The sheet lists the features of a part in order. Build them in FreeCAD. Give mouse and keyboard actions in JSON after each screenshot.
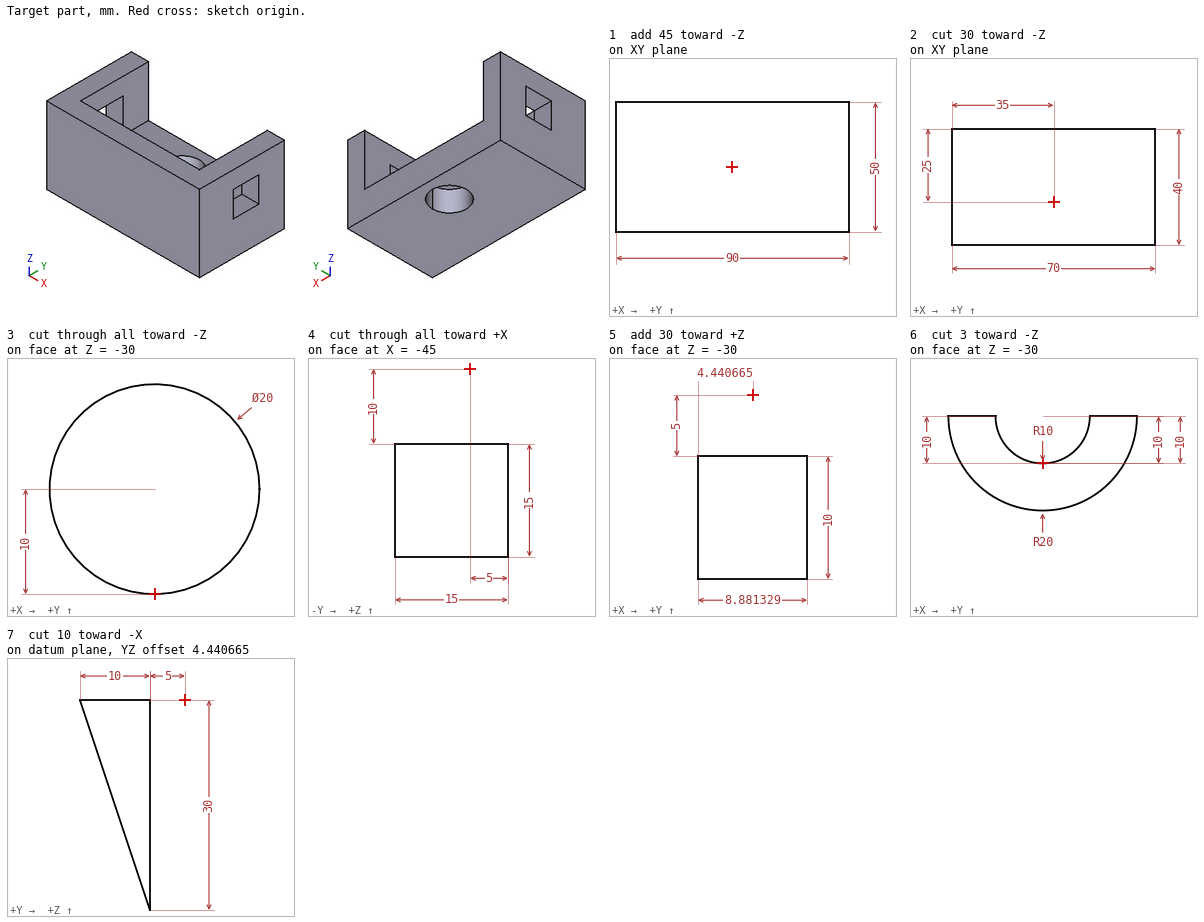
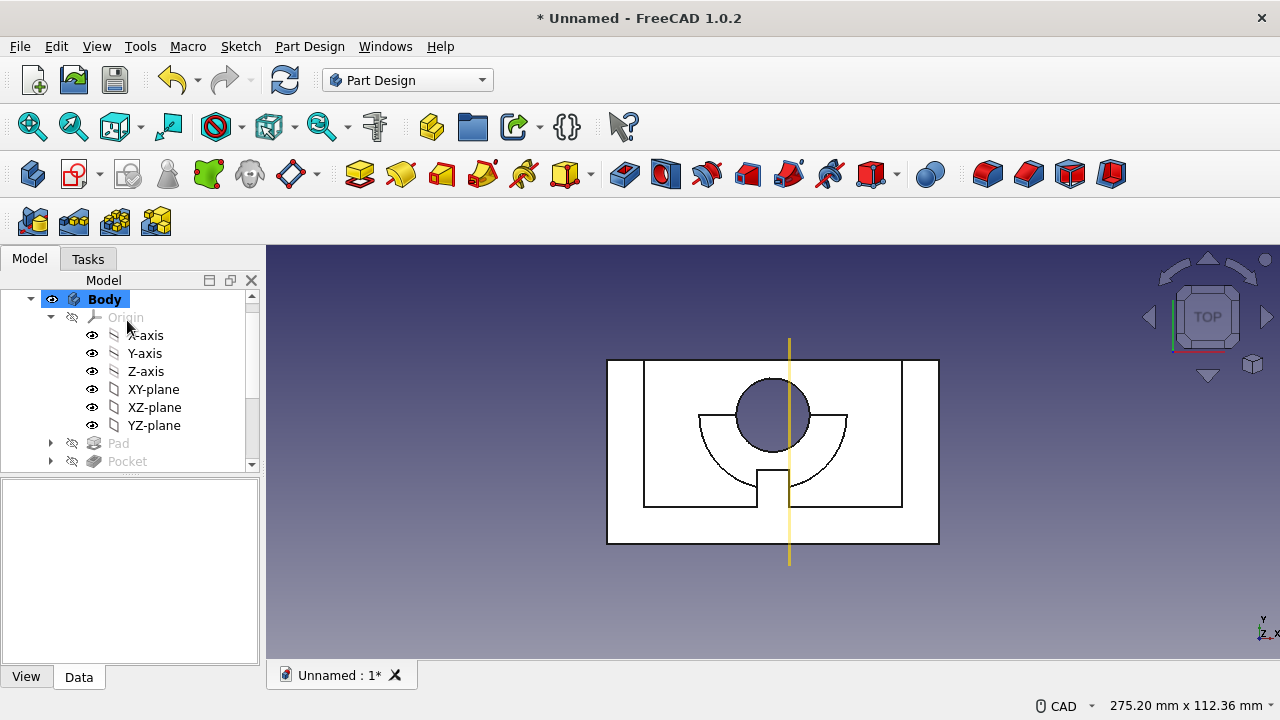
{"action": "scroll", "coordinate": [121, 385], "scroll_direction": "down", "scroll_amount": 3}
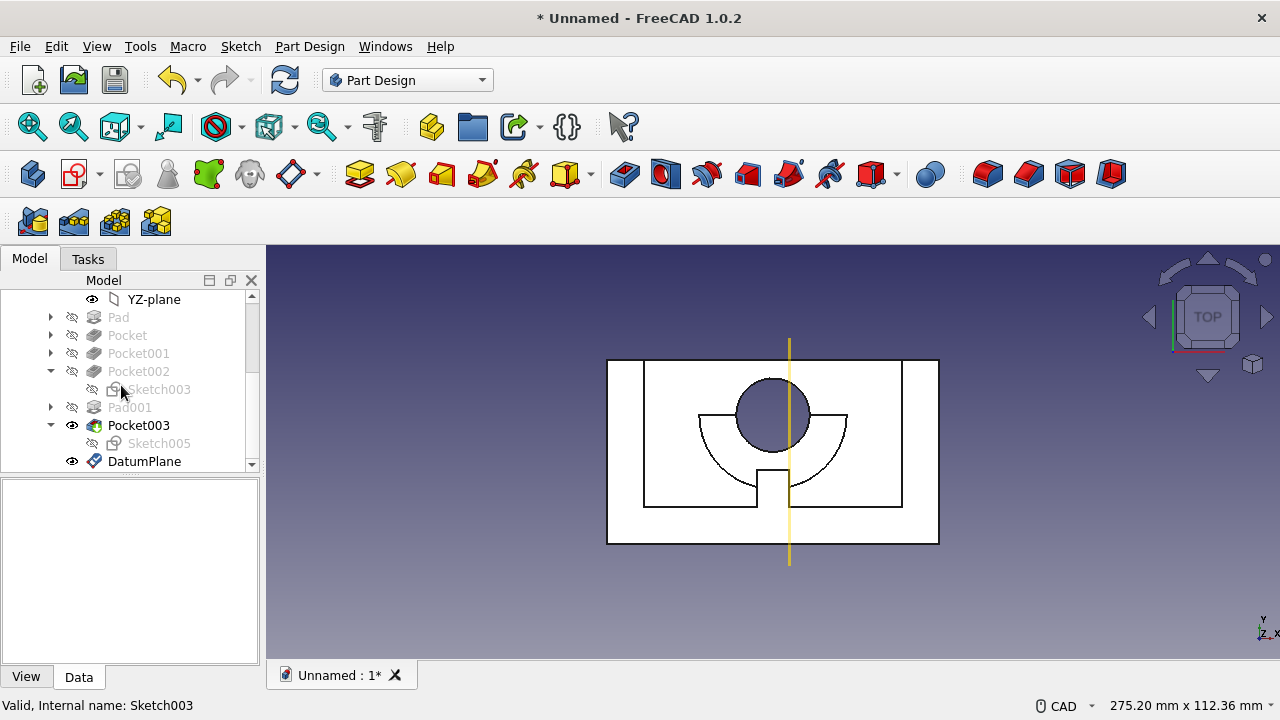
{"action": "left_click", "coordinate": [117, 461]}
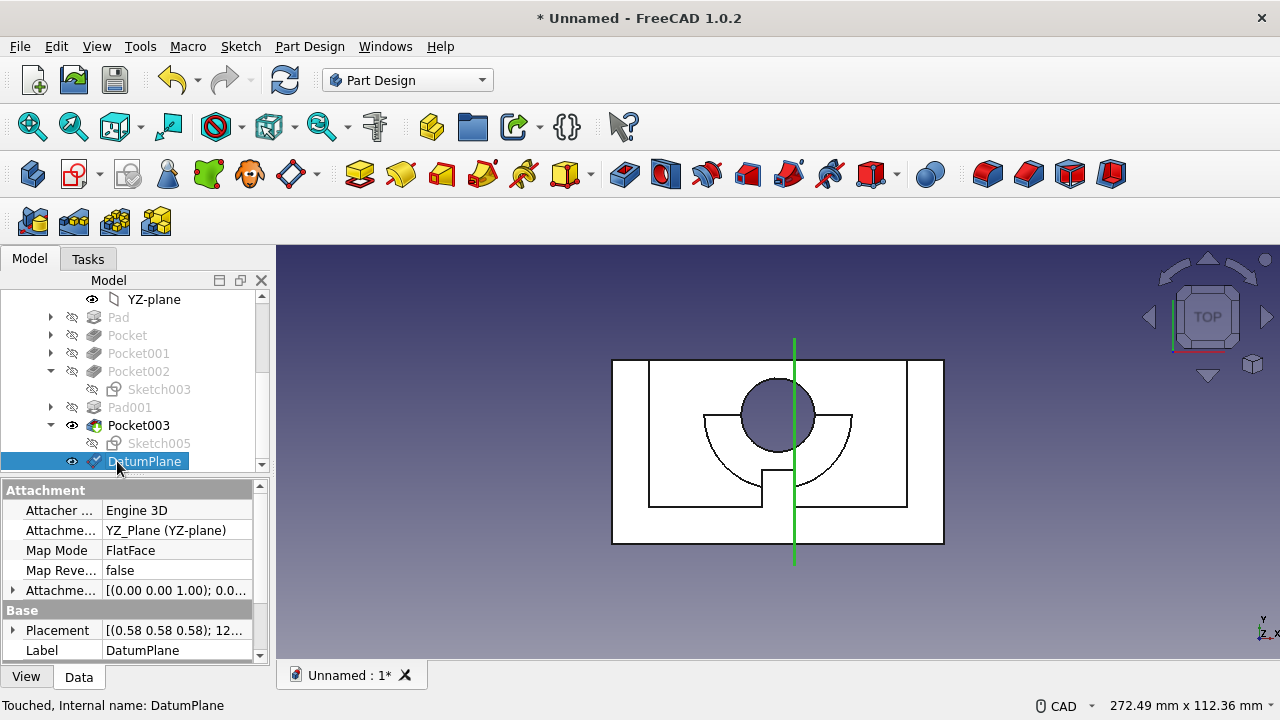
{"action": "left_click", "coordinate": [74, 174]}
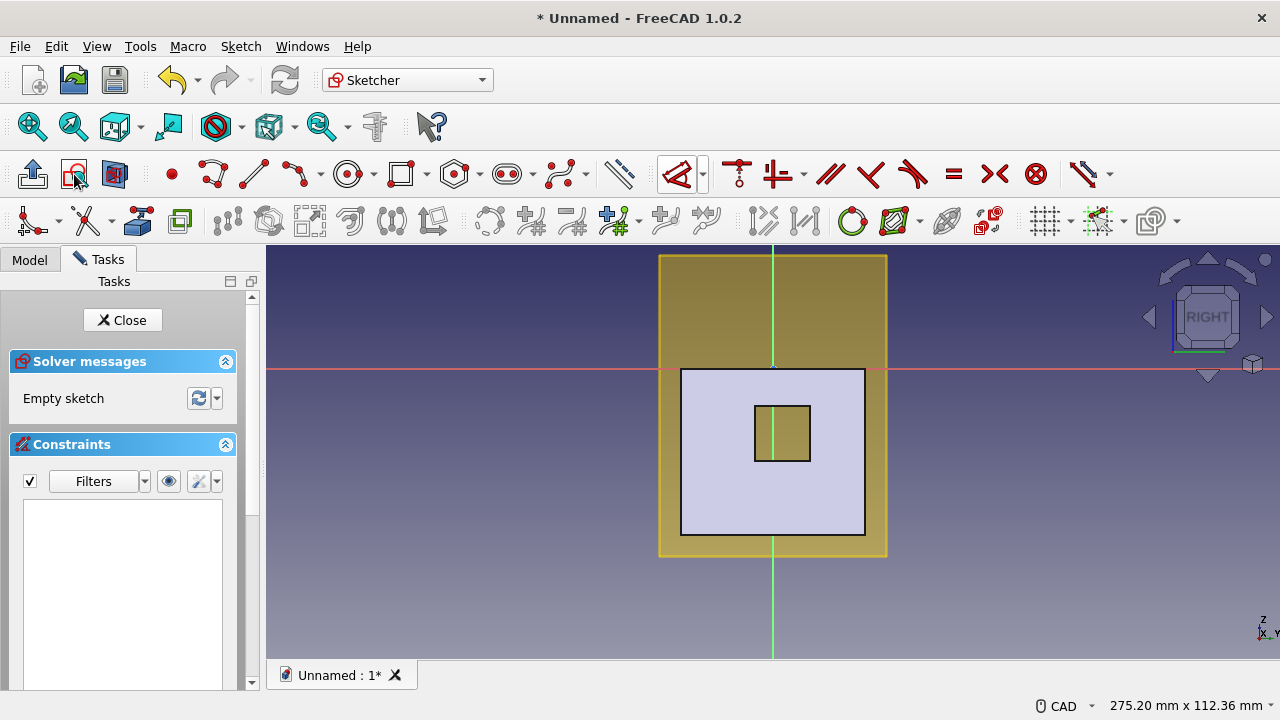
{"action": "key", "text": "q s"}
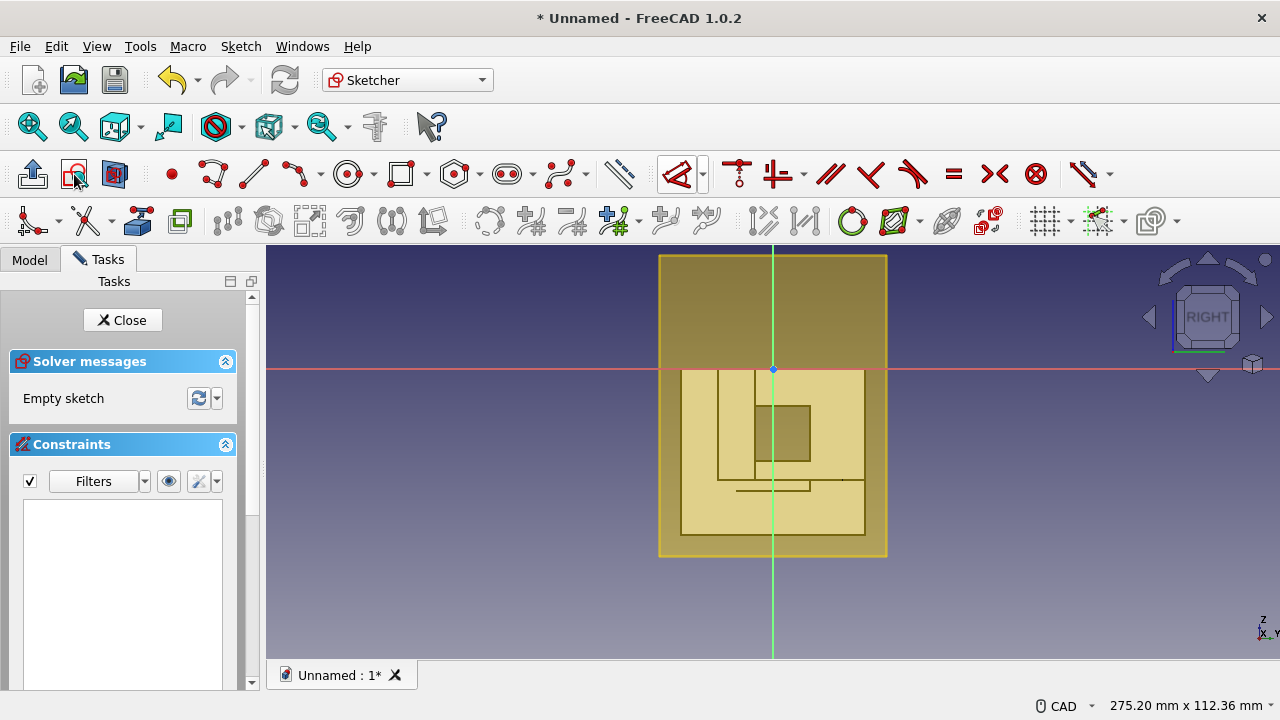
{"action": "scroll", "coordinate": [779, 402], "scroll_direction": "up", "scroll_amount": 4}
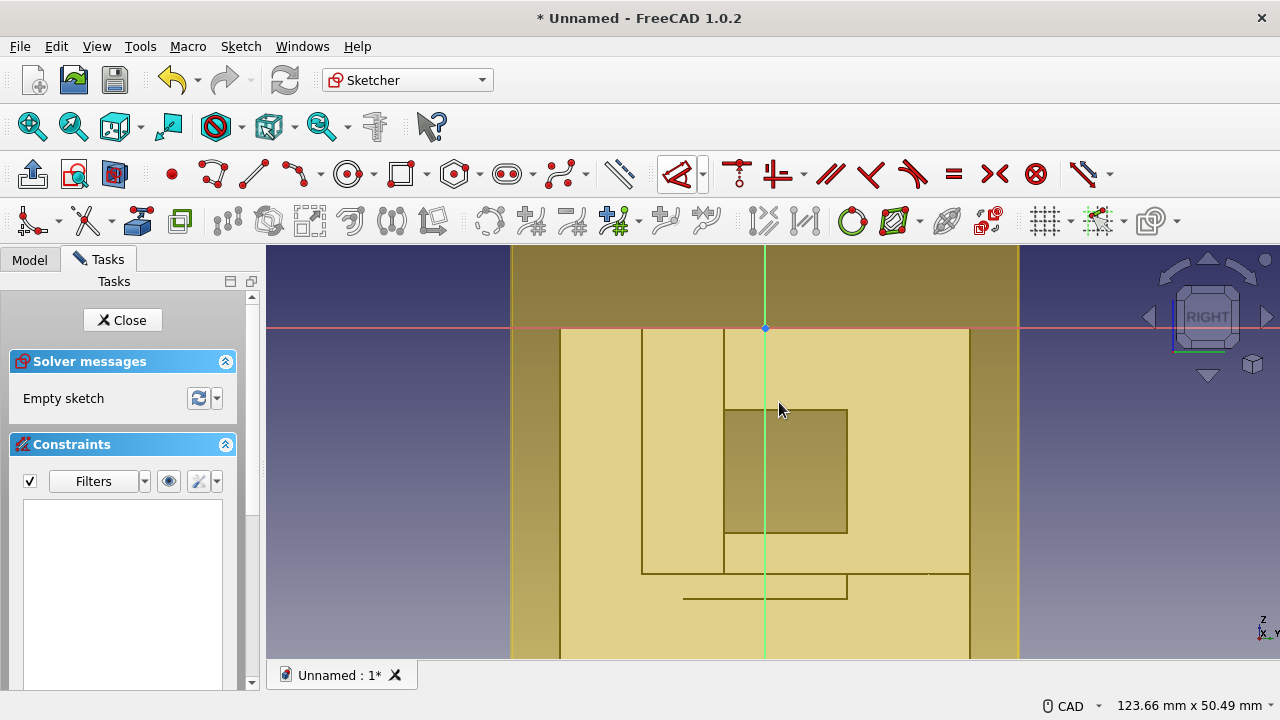
{"action": "key", "text": "g m"}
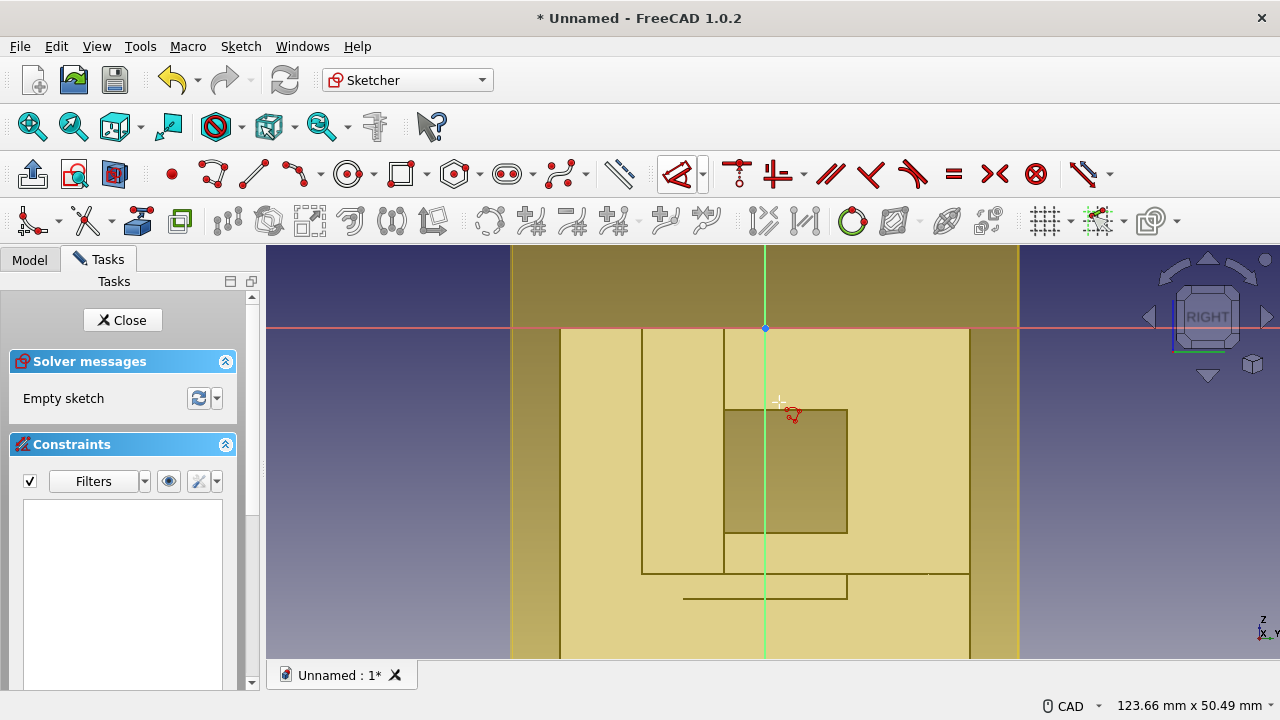
{"action": "left_click", "coordinate": [724, 328]}
{"action": "left_click", "coordinate": [642, 337]}
{"action": "left_click", "coordinate": [724, 574]}
{"action": "left_click", "coordinate": [724, 328]}
{"action": "key", "text": "Escape"}
{"action": "key", "text": "Escape"}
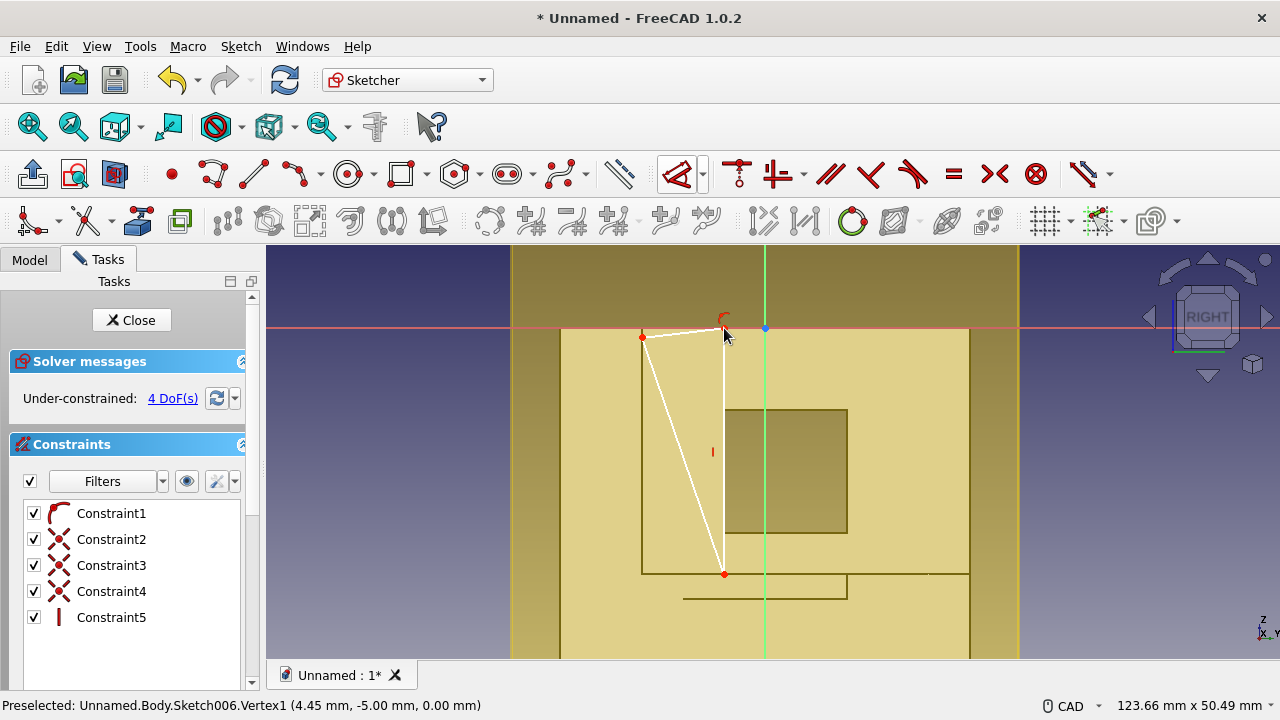
{"action": "left_click", "coordinate": [699, 331]}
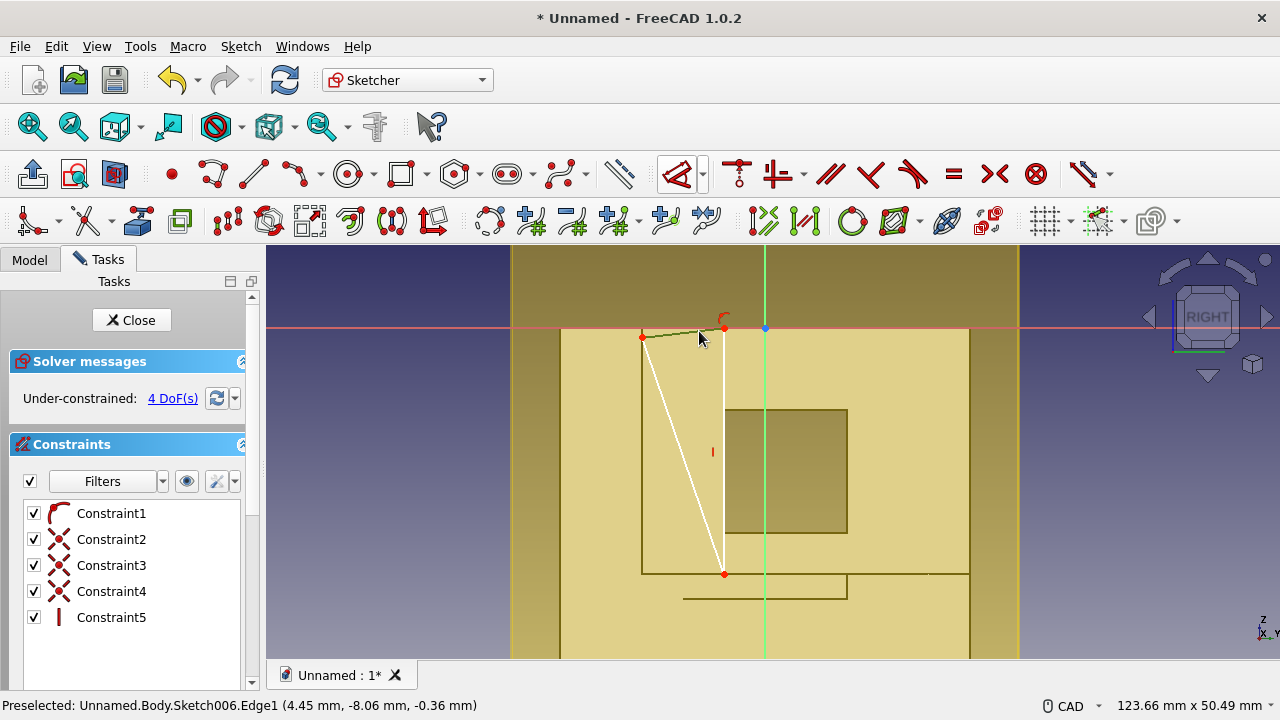
{"action": "key", "text": "h"}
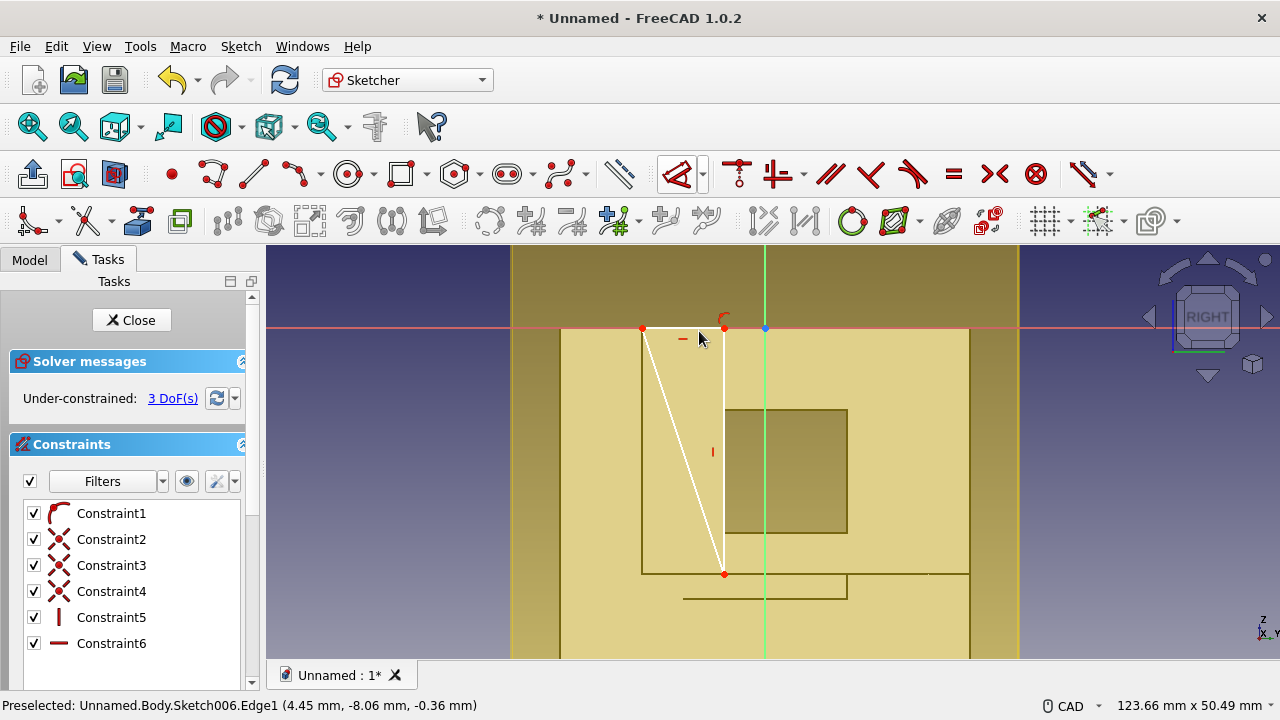
{"action": "left_click", "coordinate": [699, 328]}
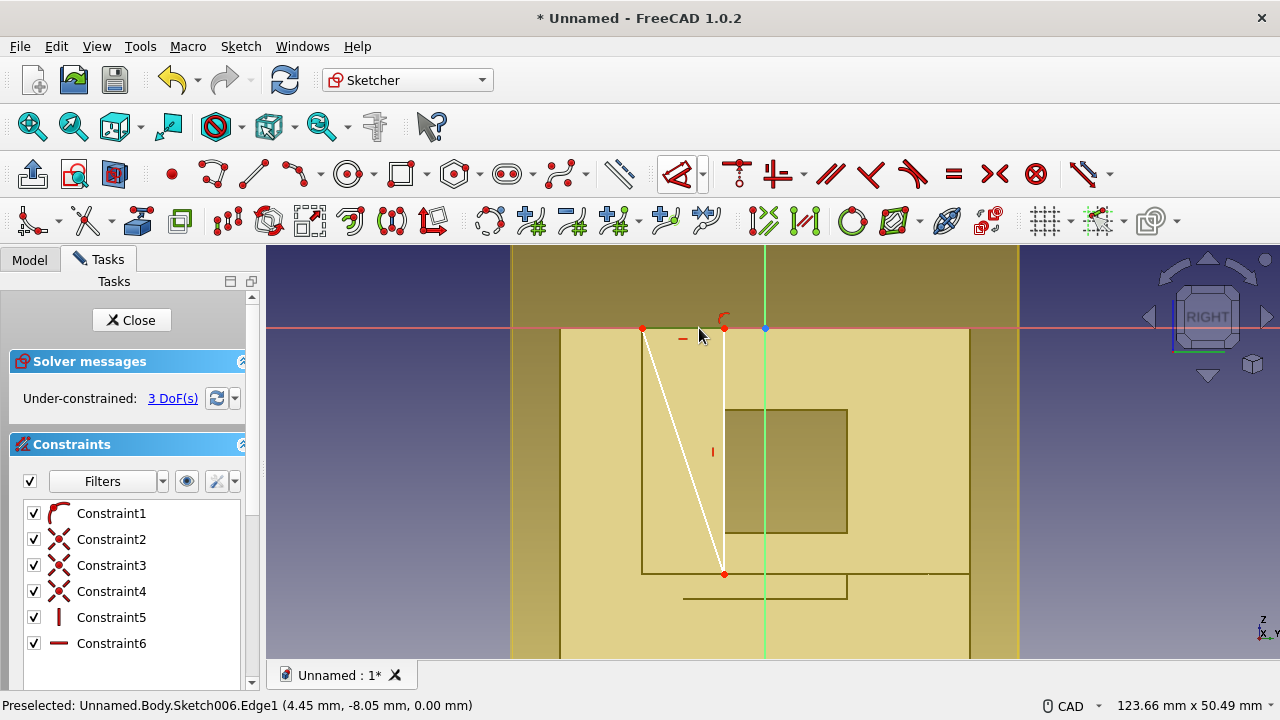
{"action": "key", "text": "l"}